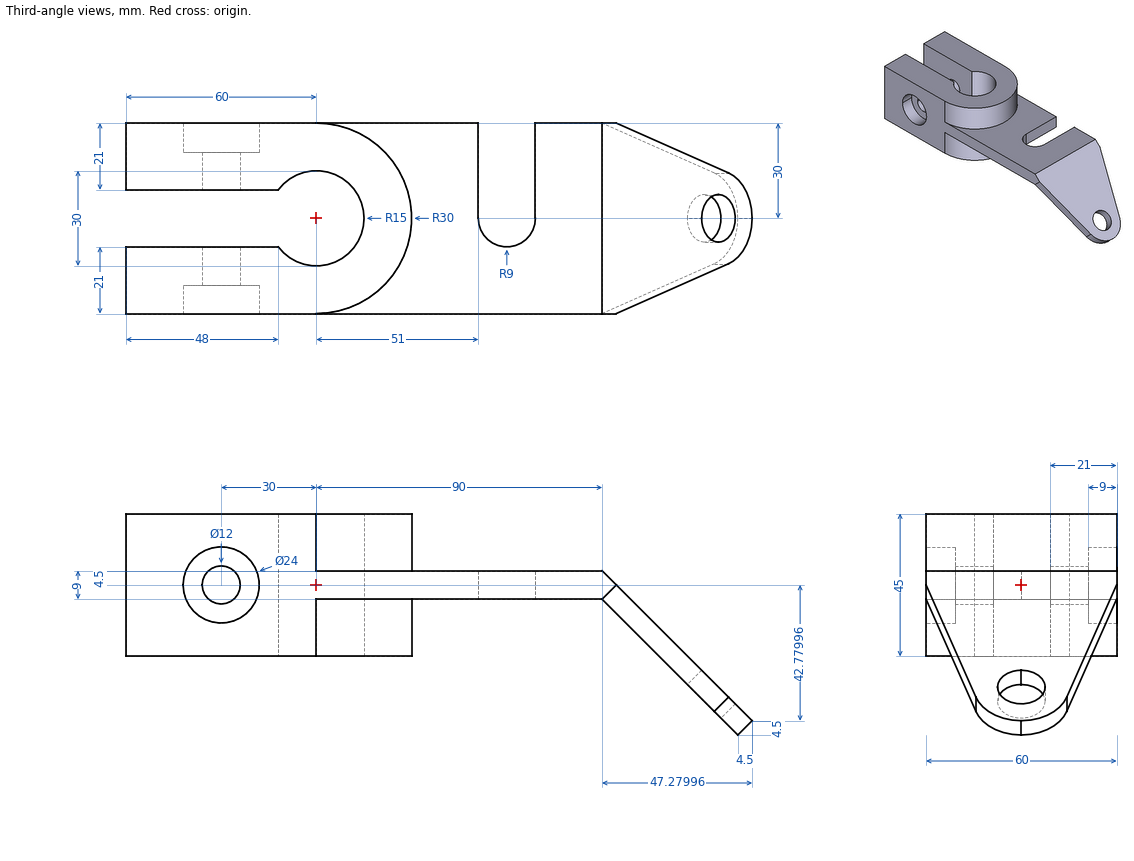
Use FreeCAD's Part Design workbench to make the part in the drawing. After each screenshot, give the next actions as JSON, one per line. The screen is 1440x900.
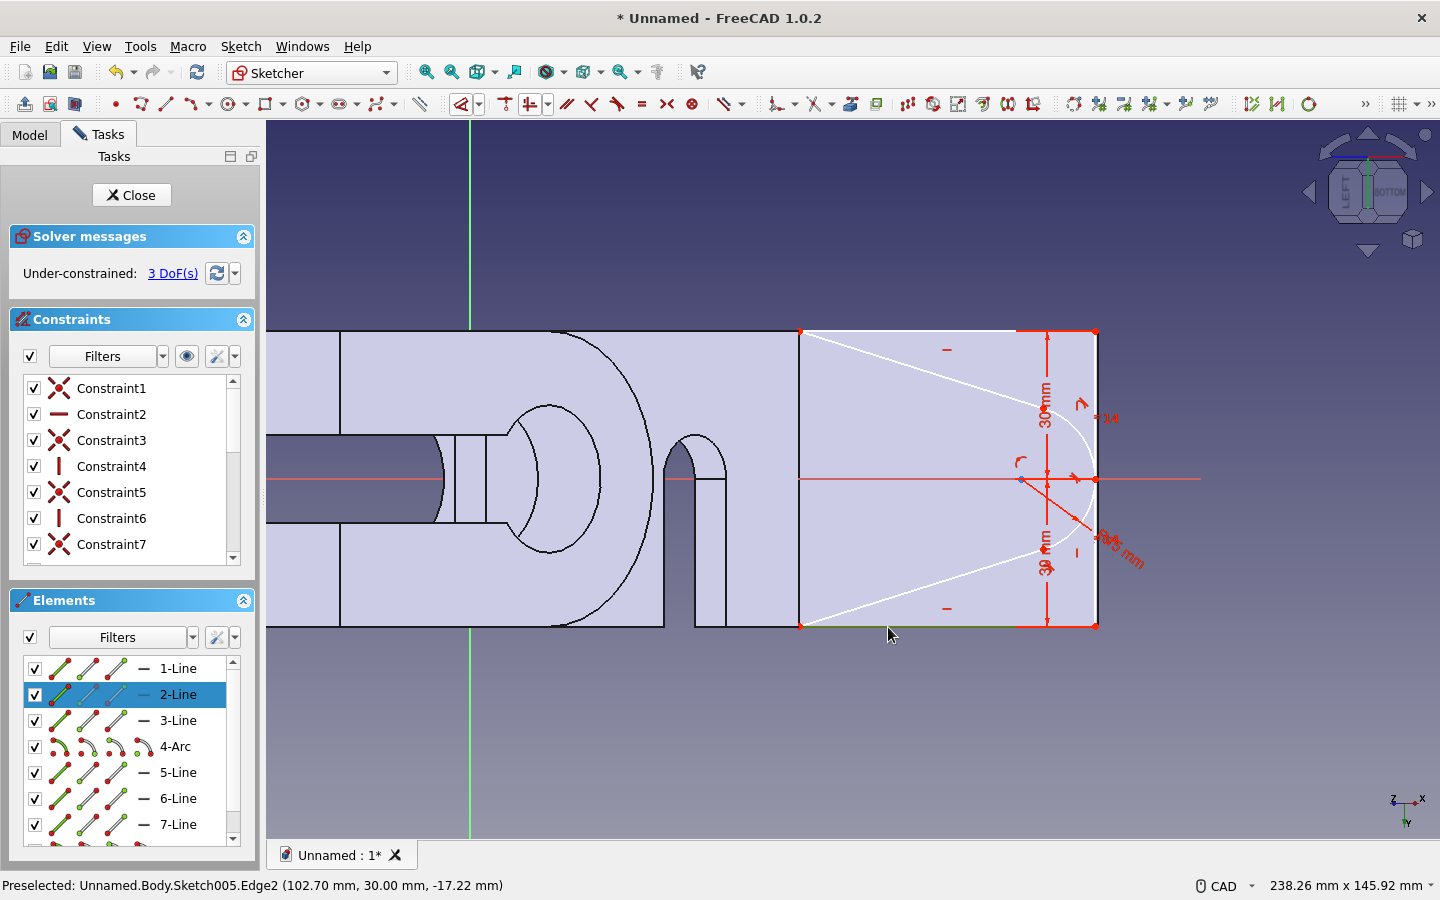
{"action": "left_click", "coordinate": [478, 104]}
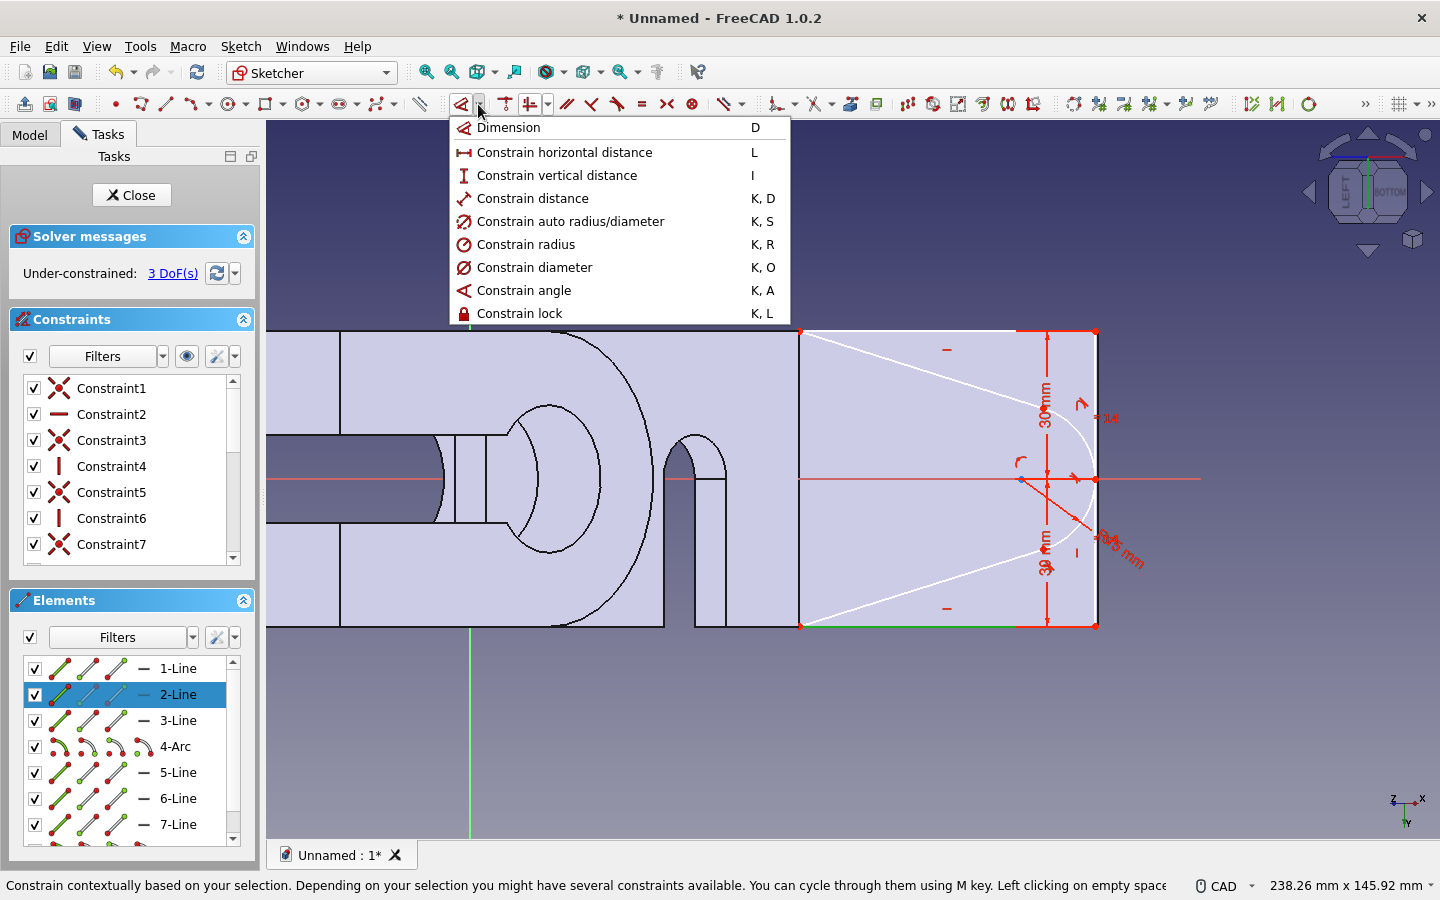
{"action": "left_click", "coordinate": [620, 152]}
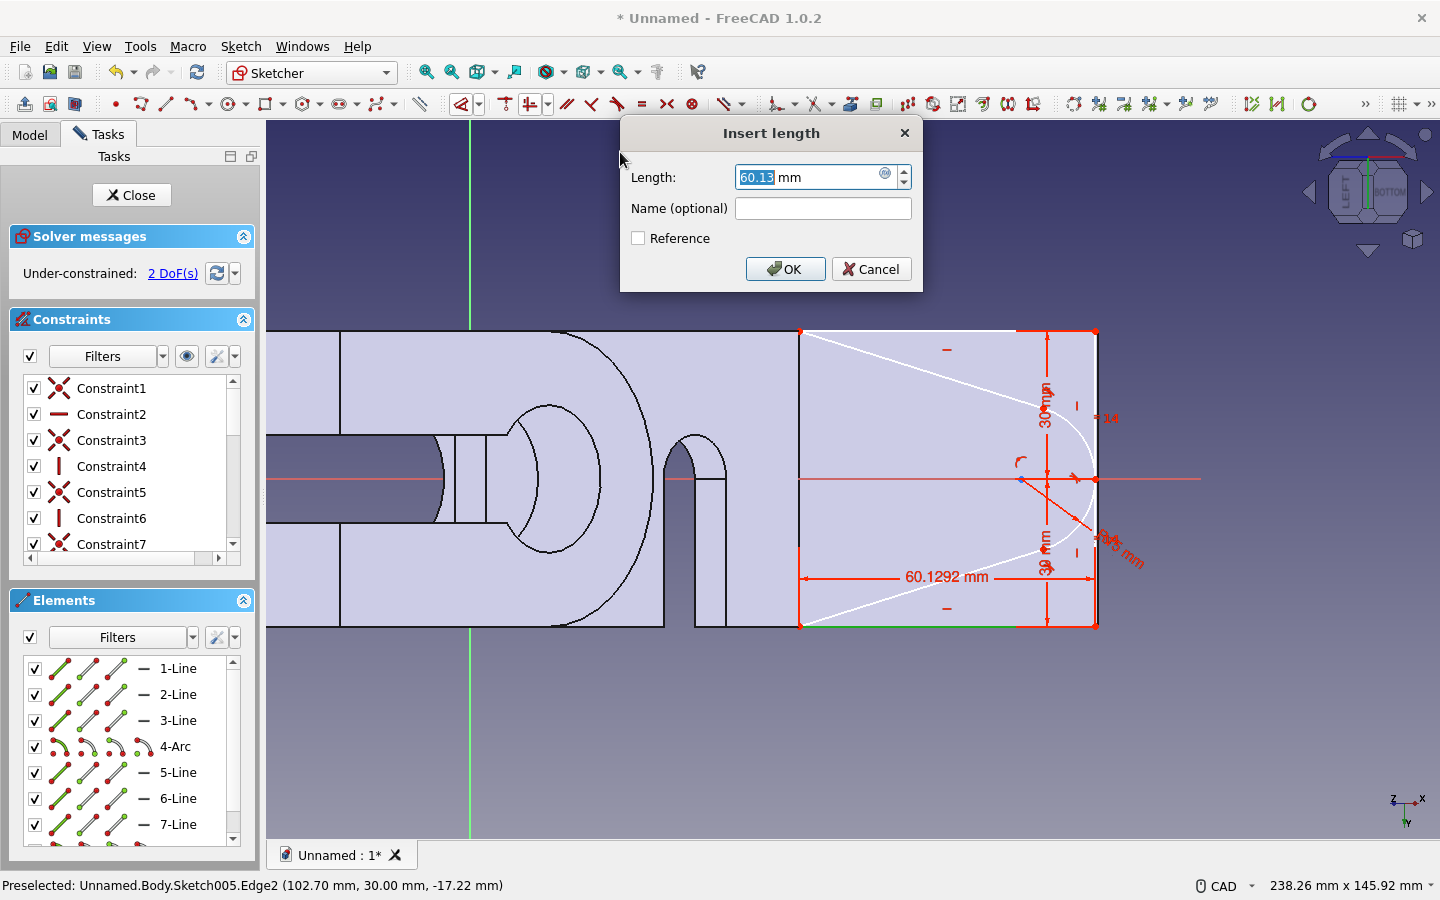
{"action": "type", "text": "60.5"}
{"action": "key", "text": "Return"}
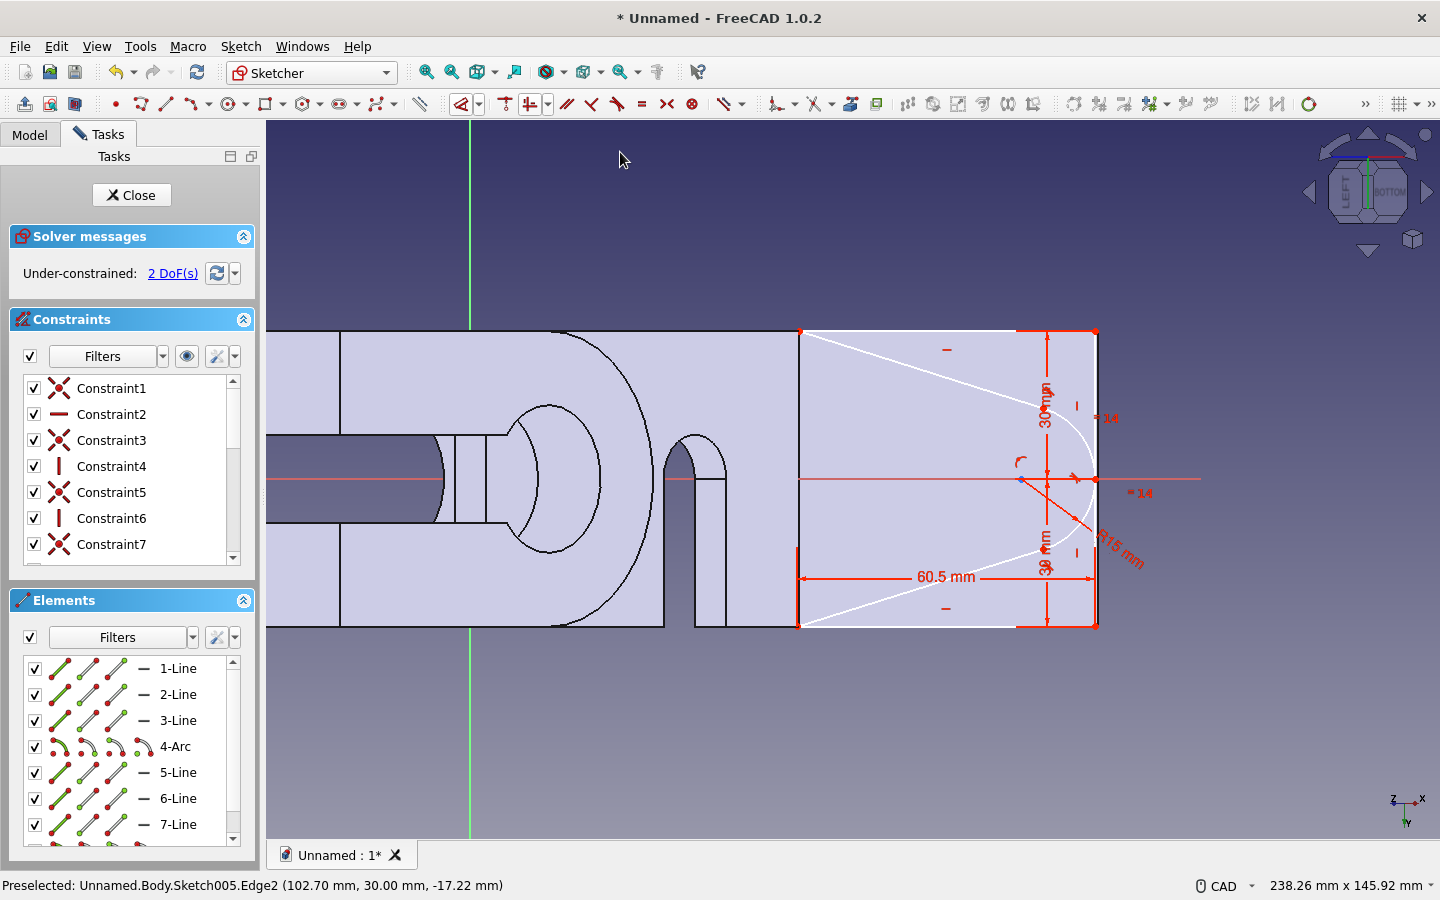
{"action": "left_click", "coordinate": [1006, 331]}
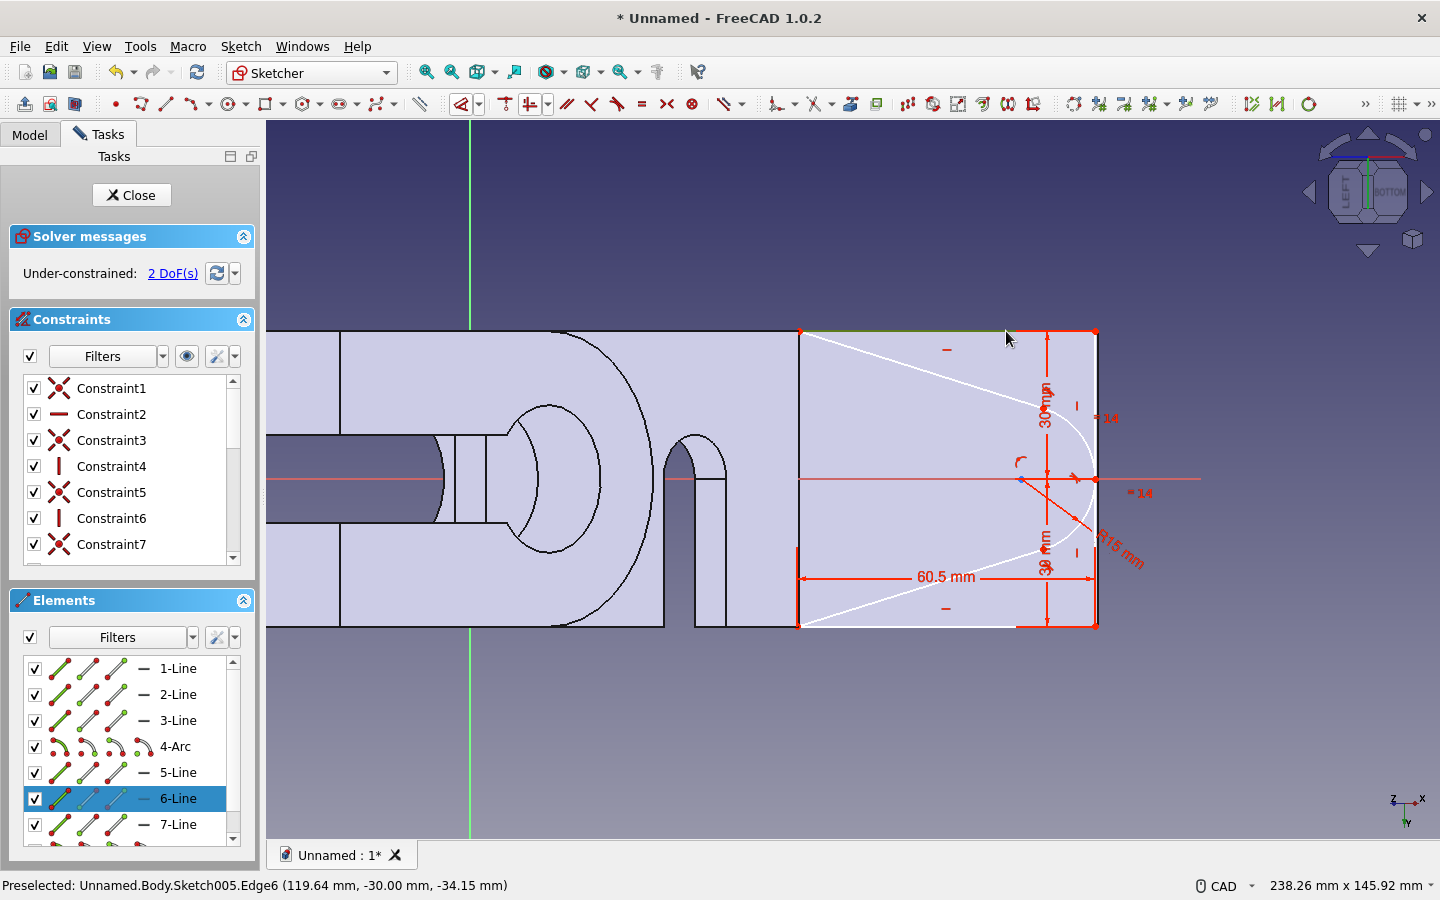
{"action": "key", "text": "l"}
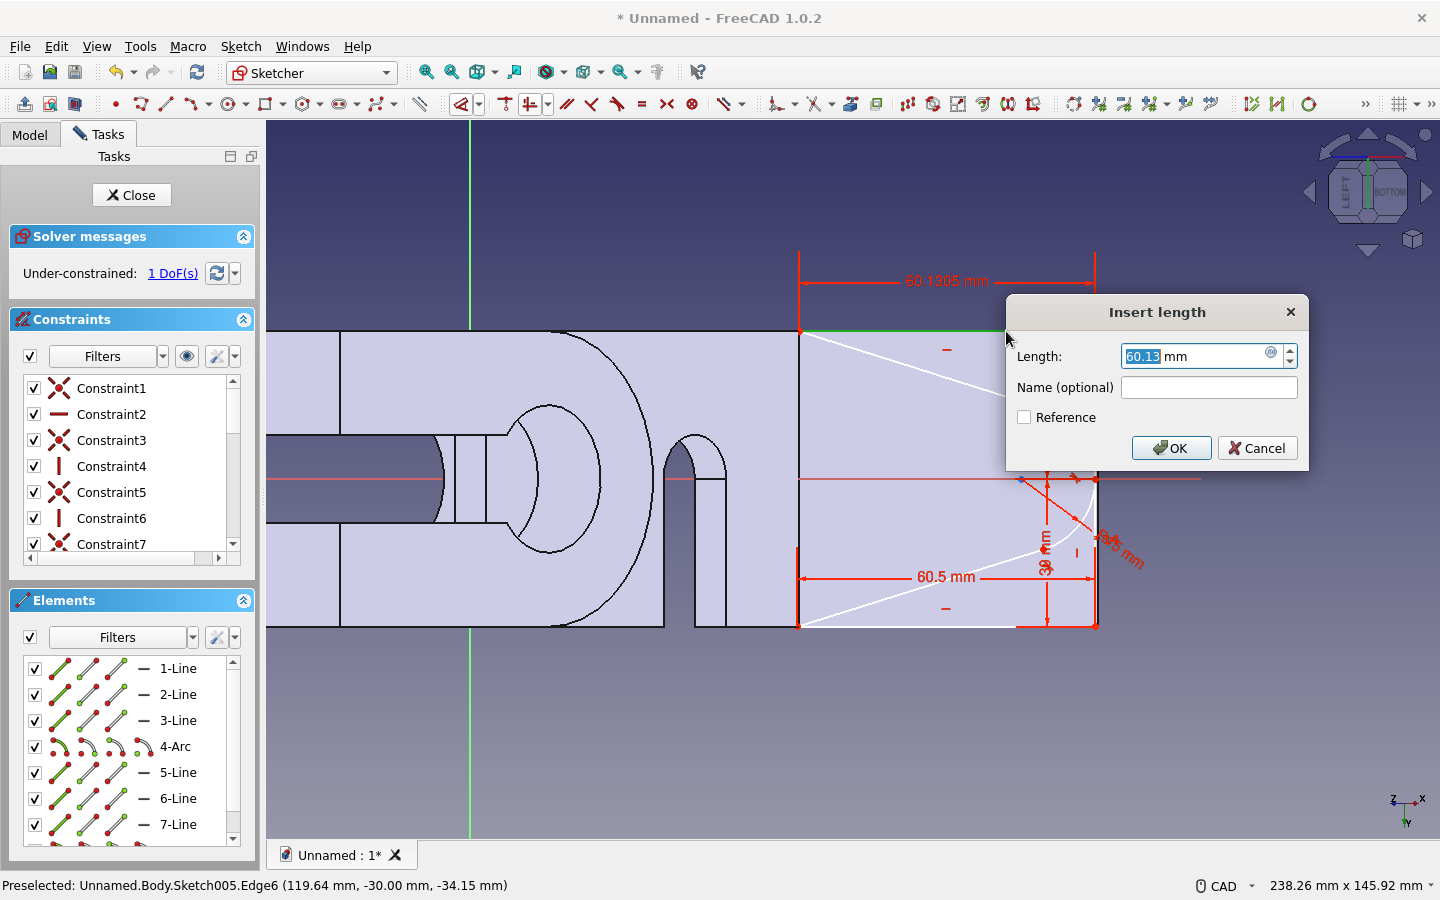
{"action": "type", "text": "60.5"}
{"action": "key", "text": "Return"}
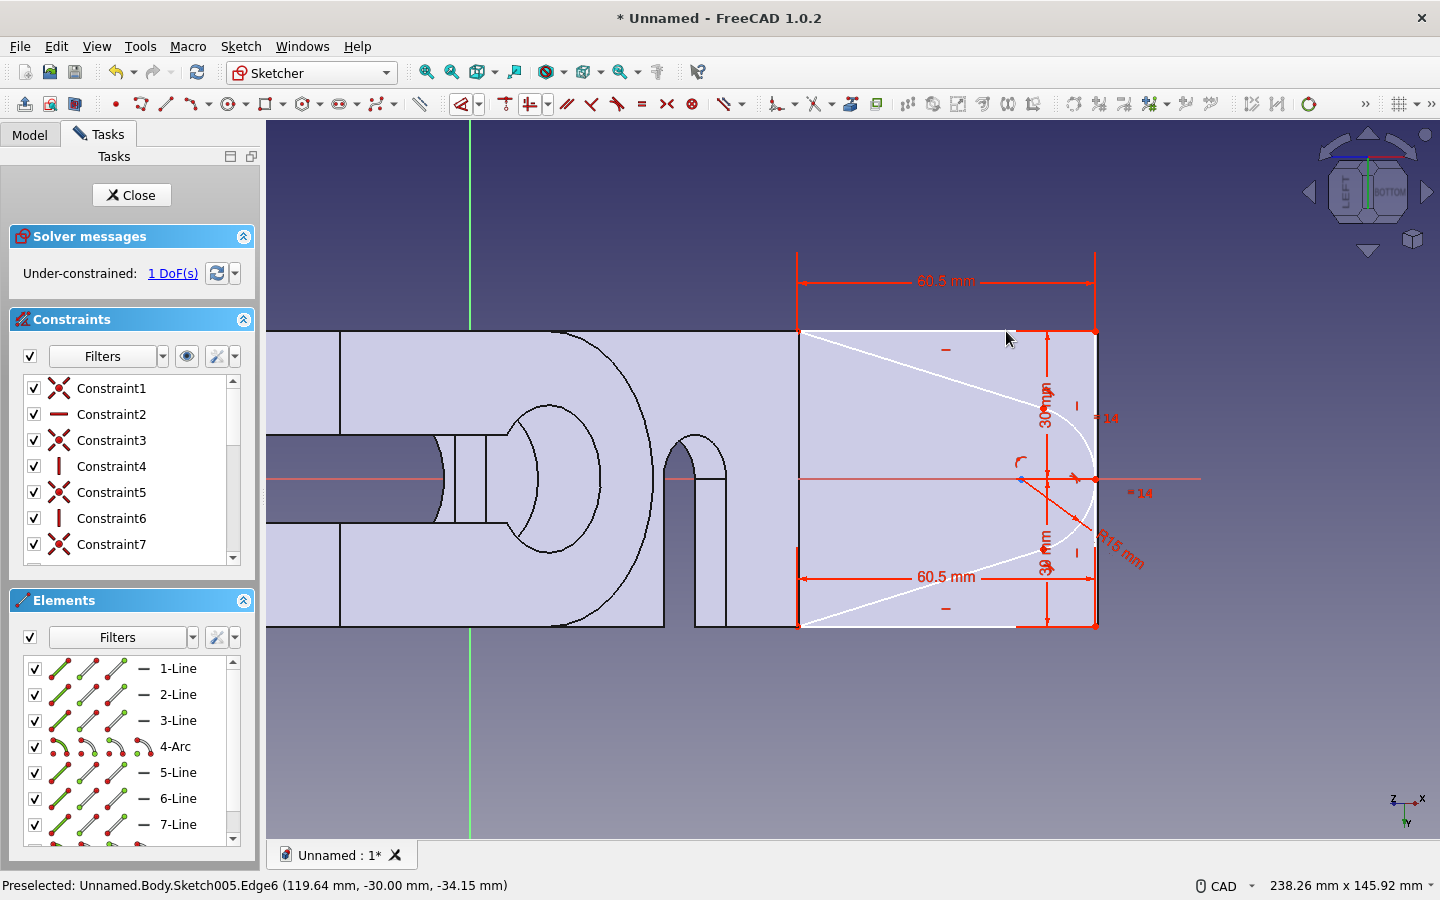
{"action": "left_click", "coordinate": [1044, 550]}